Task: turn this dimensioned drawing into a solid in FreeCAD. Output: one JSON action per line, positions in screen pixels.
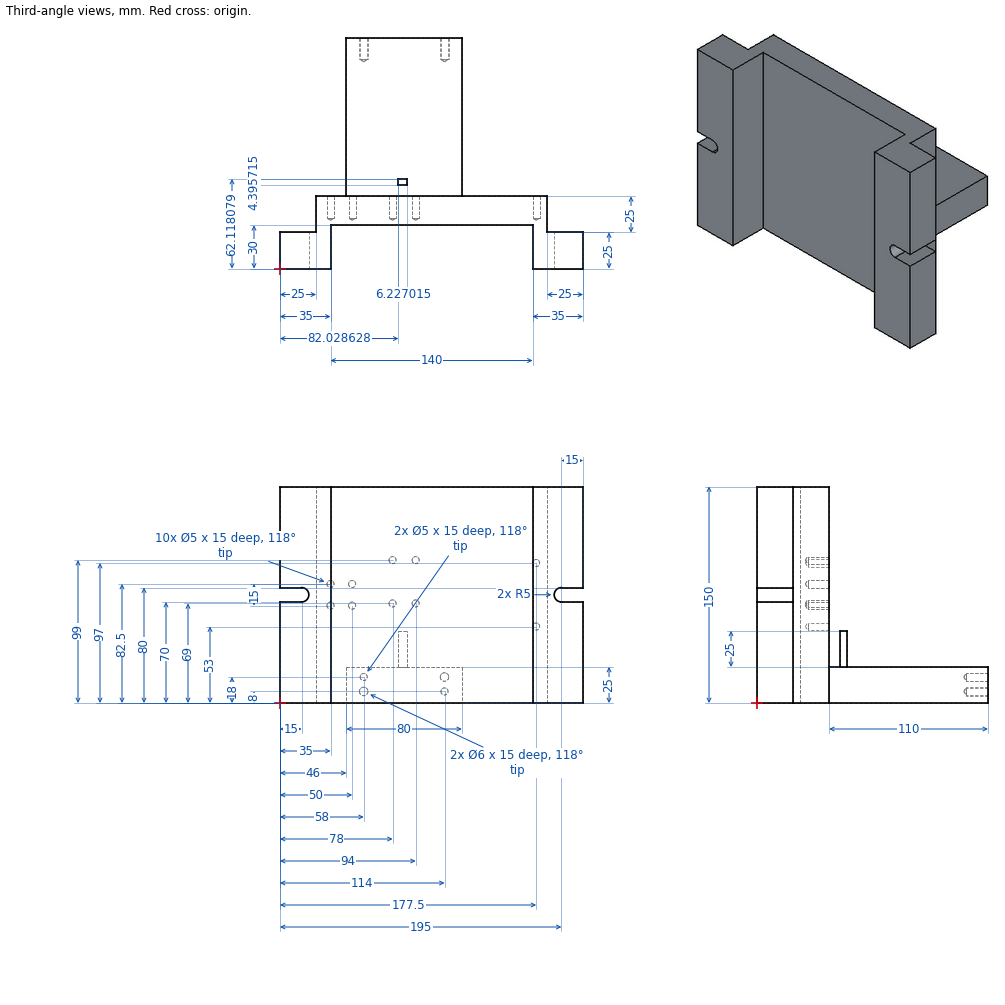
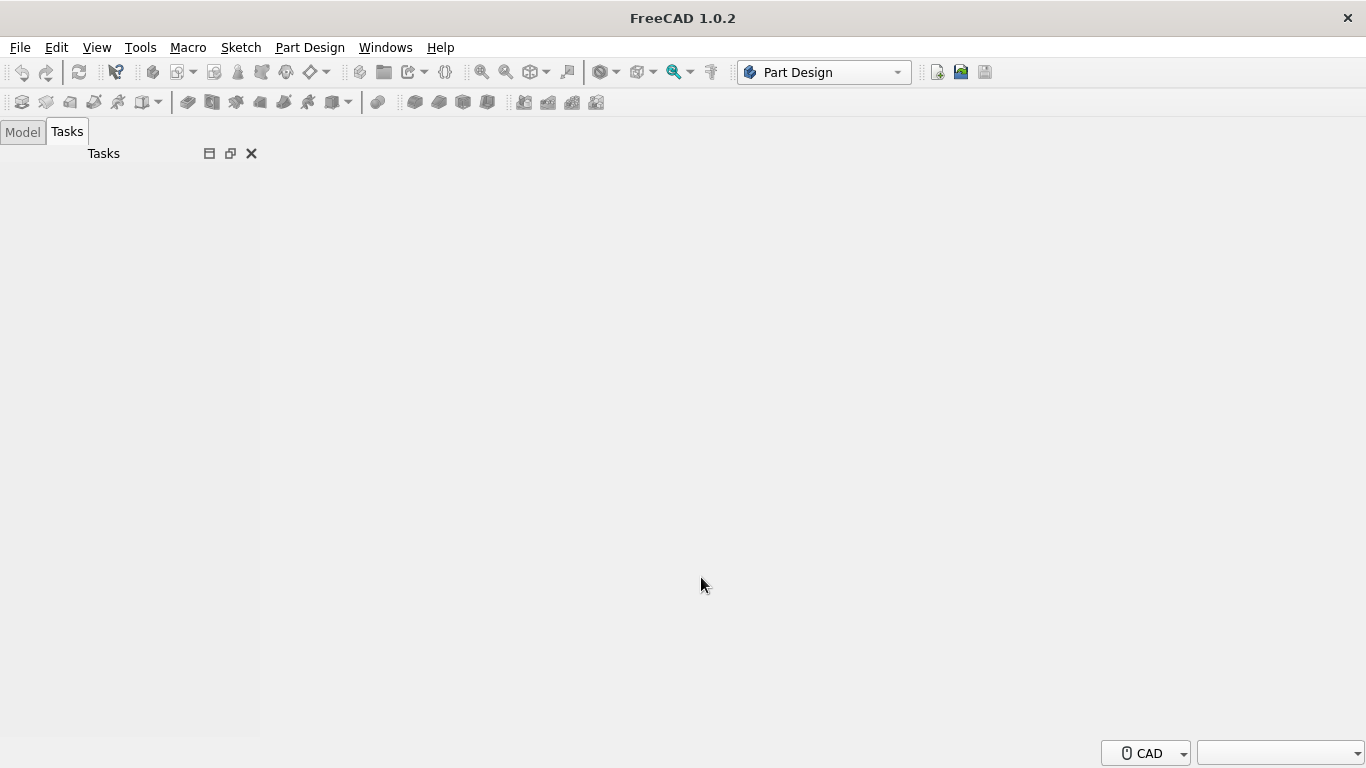
{"action": "key", "text": "ctrl+n"}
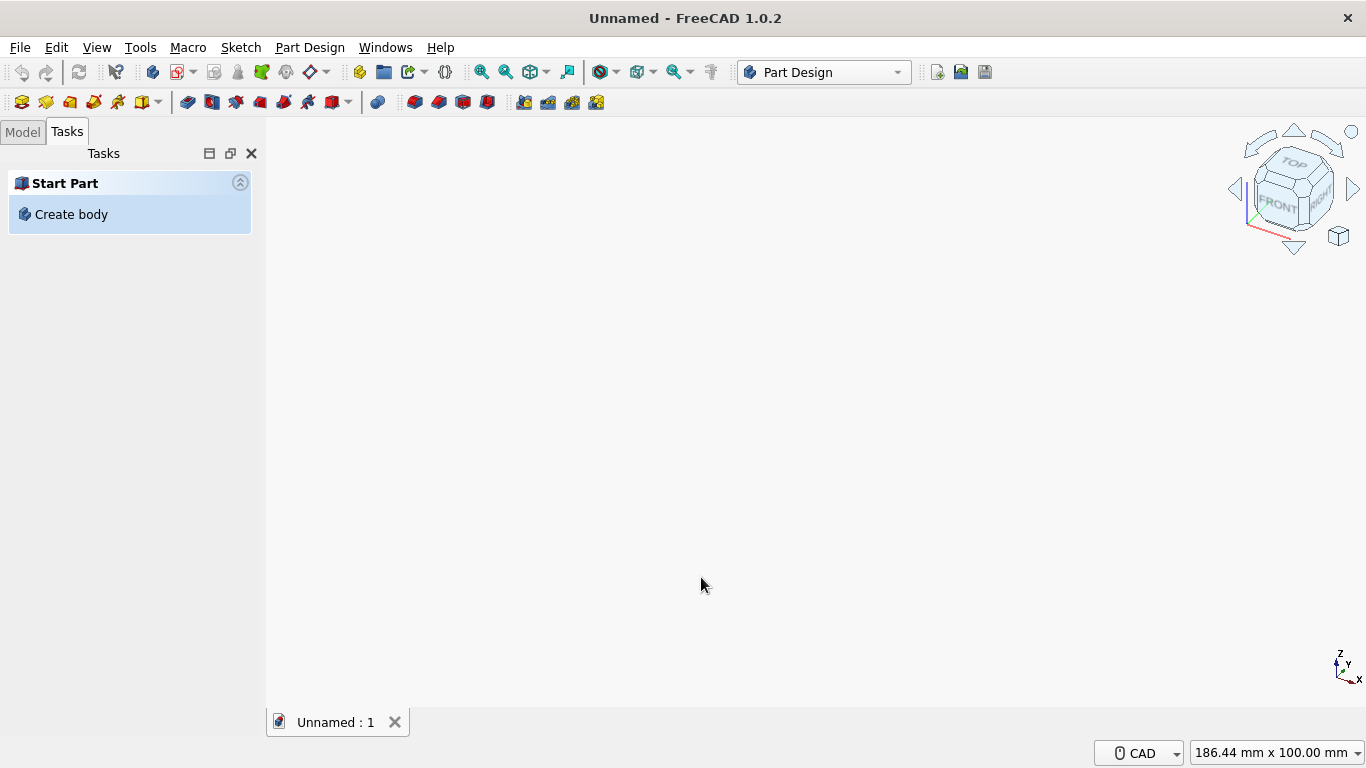
{"action": "left_click", "coordinate": [178, 72]}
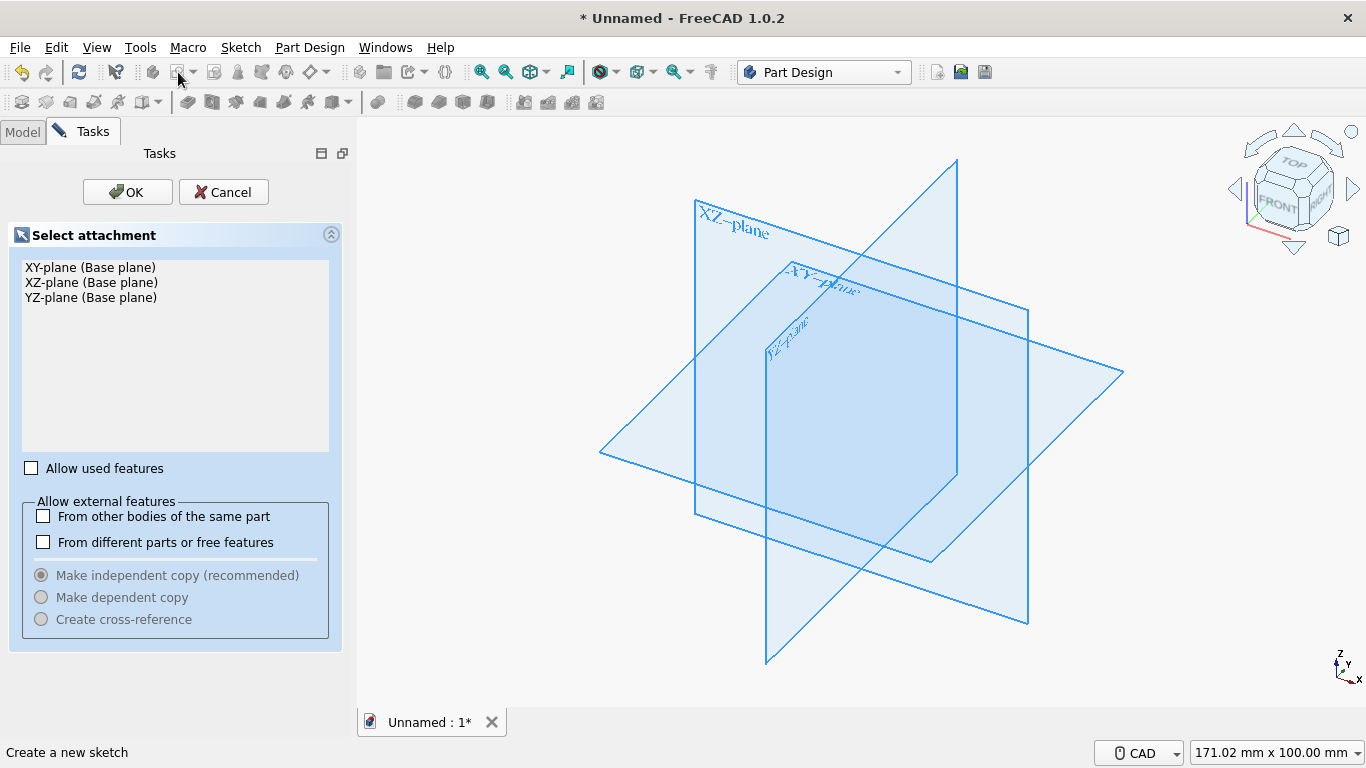
{"action": "left_click", "coordinate": [82, 268]}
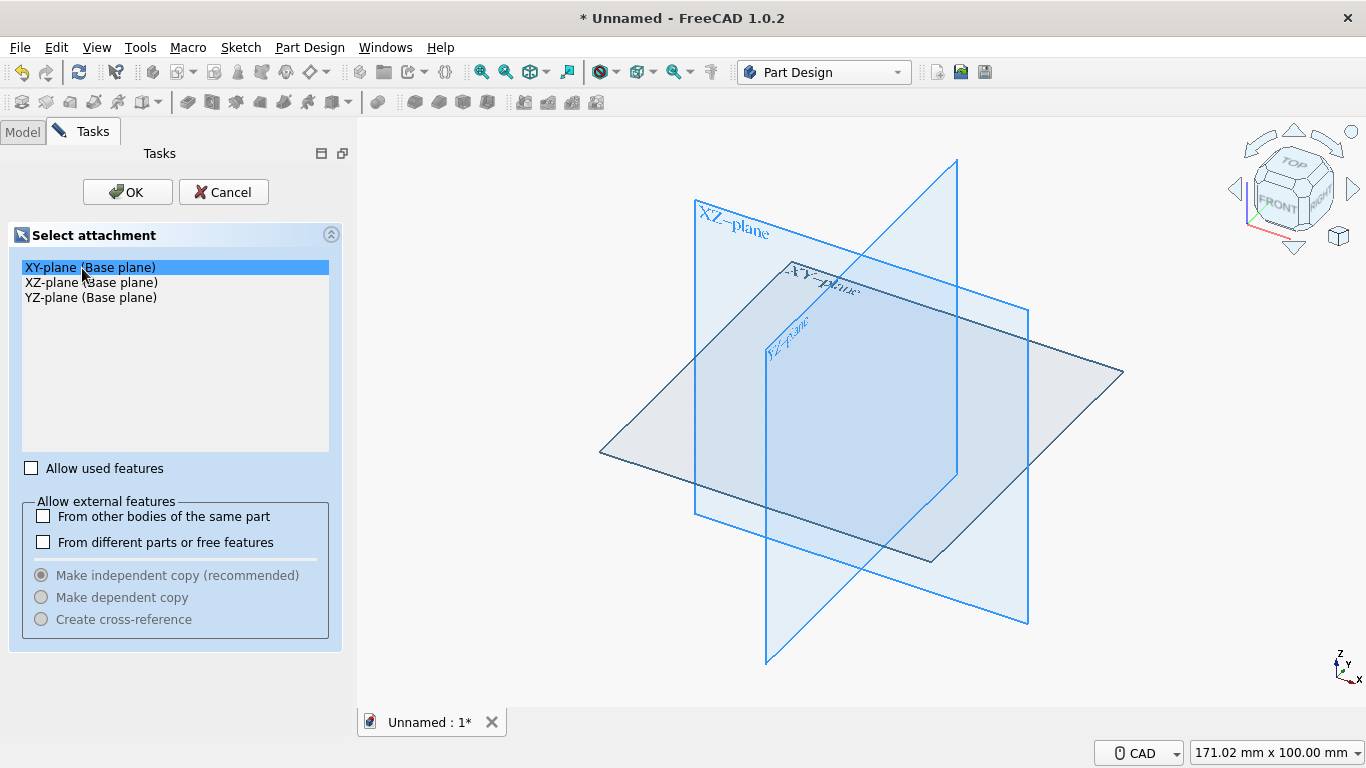
{"action": "left_click", "coordinate": [128, 192]}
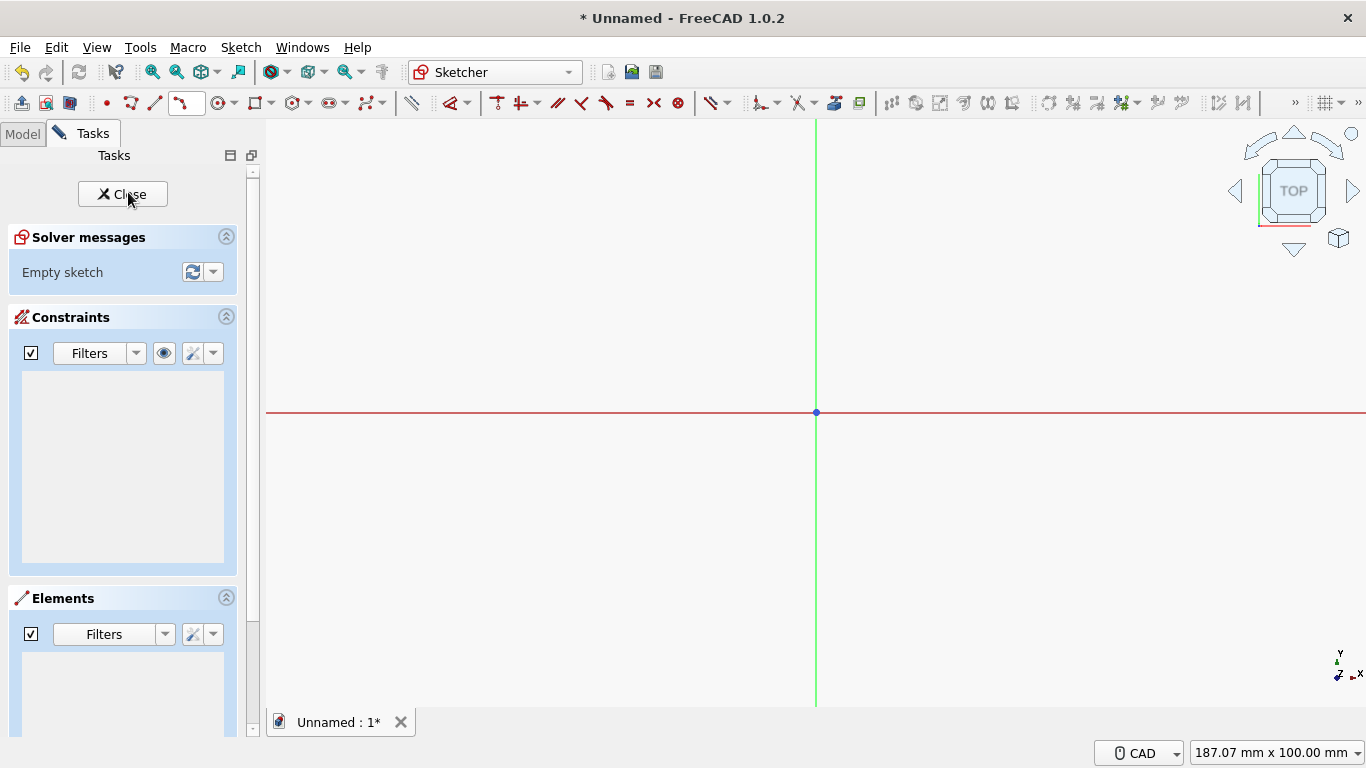
{"action": "scroll", "coordinate": [294, 533], "scroll_direction": "down", "scroll_amount": 4}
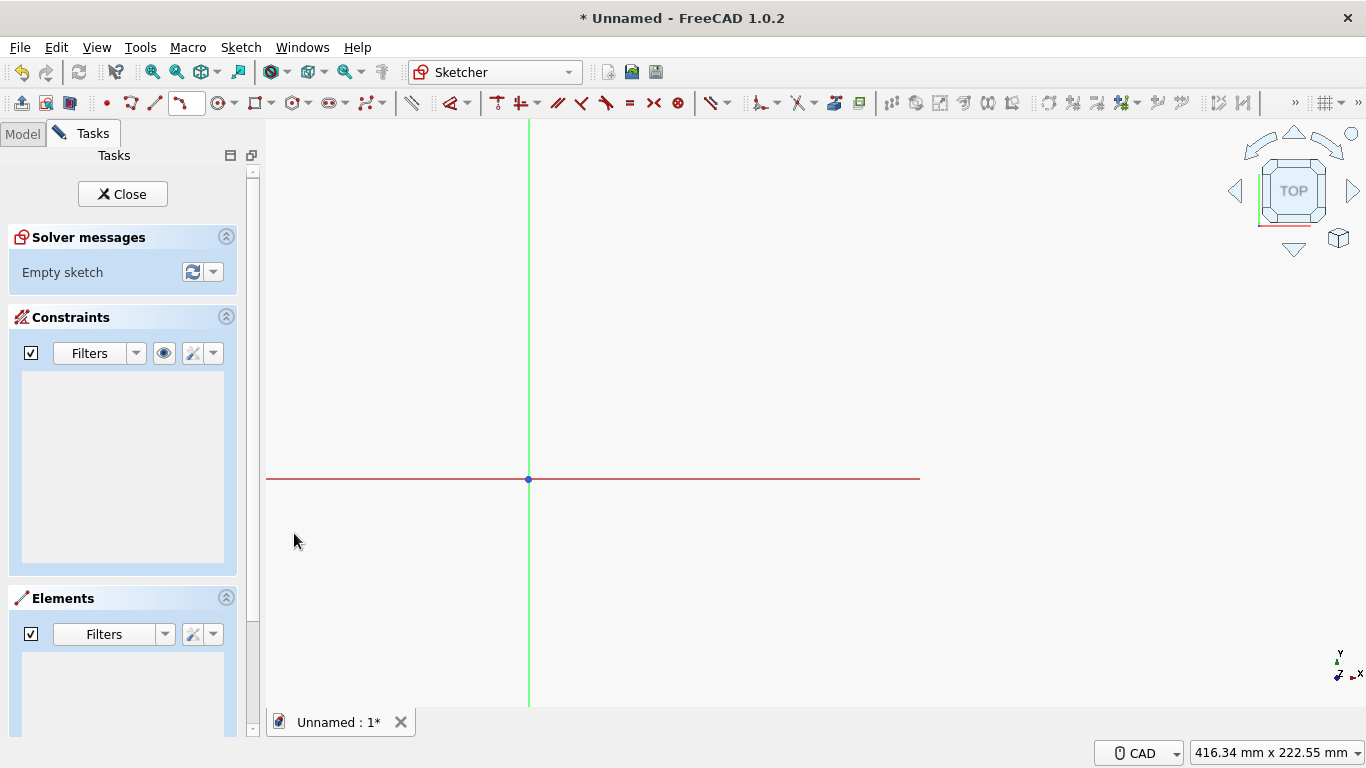
{"action": "key", "text": "g m"}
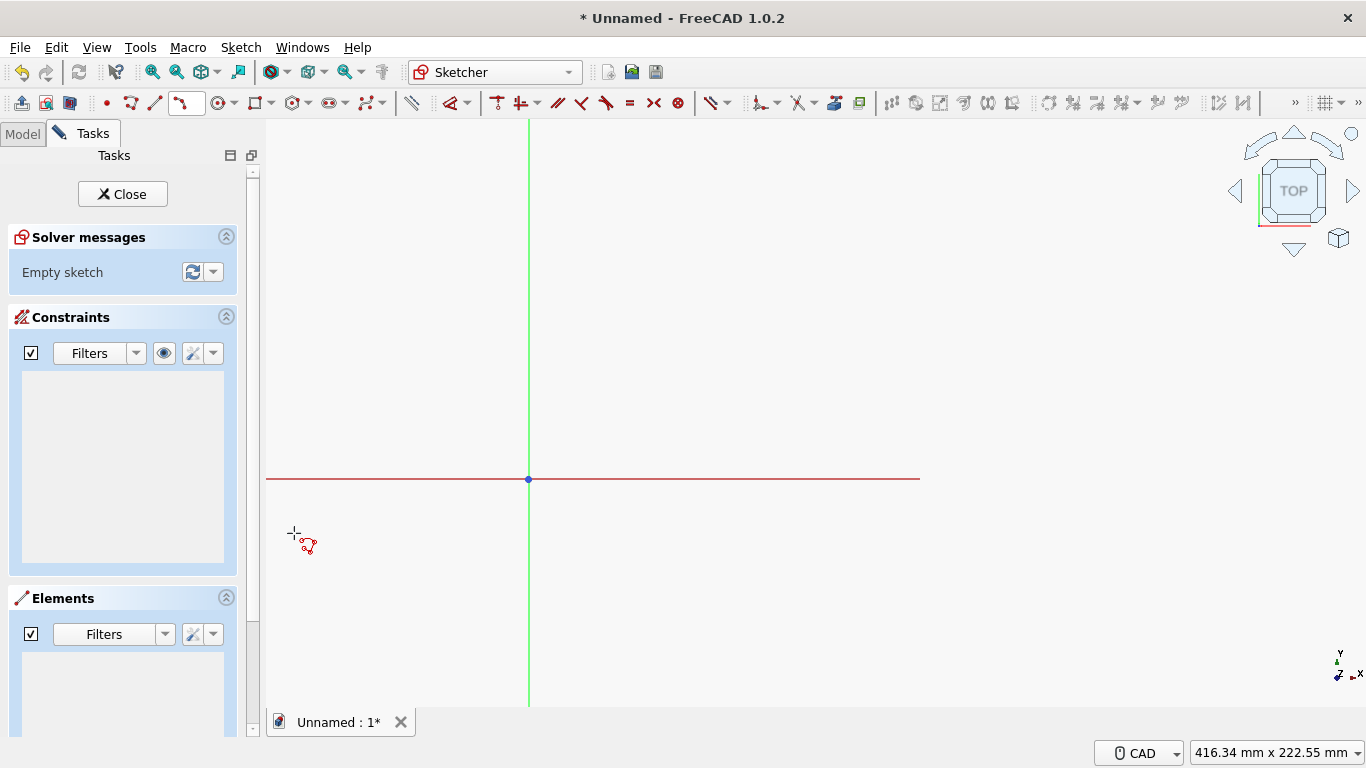
{"action": "left_click", "coordinate": [529, 479]}
{"action": "left_click", "coordinate": [621, 470]}
{"action": "left_click", "coordinate": [621, 400]}
{"action": "left_click", "coordinate": [991, 400]}
{"action": "left_click", "coordinate": [991, 479]}
{"action": "left_click", "coordinate": [1083, 470]}
{"action": "left_click", "coordinate": [1083, 413]}
{"action": "left_click", "coordinate": [1017, 413]}
{"action": "left_click", "coordinate": [1017, 347]}
{"action": "left_click", "coordinate": [595, 347]}
{"action": "left_click", "coordinate": [595, 413]}
{"action": "left_click", "coordinate": [538, 413]}
{"action": "left_click", "coordinate": [529, 479]}
{"action": "key", "text": "Escape"}
{"action": "key", "text": "Escape"}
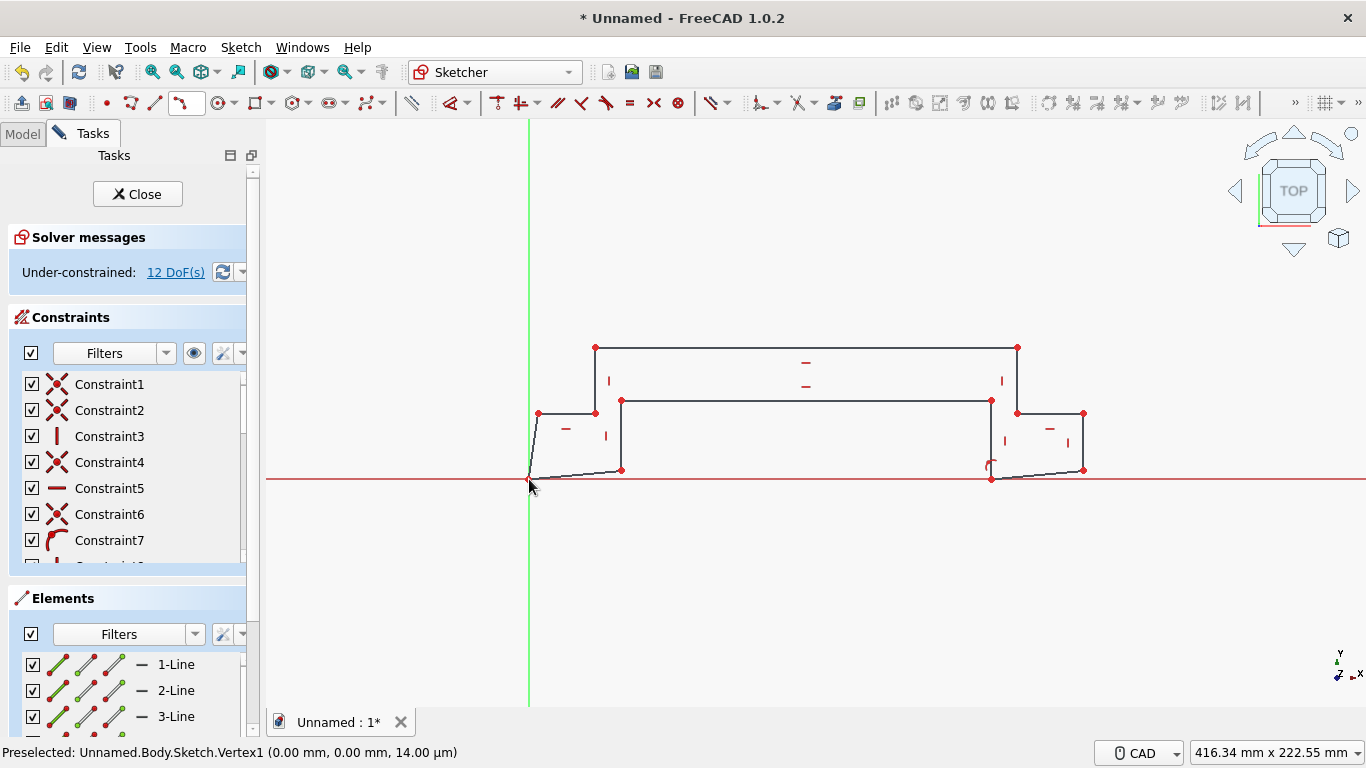
{"action": "left_click", "coordinate": [556, 477]}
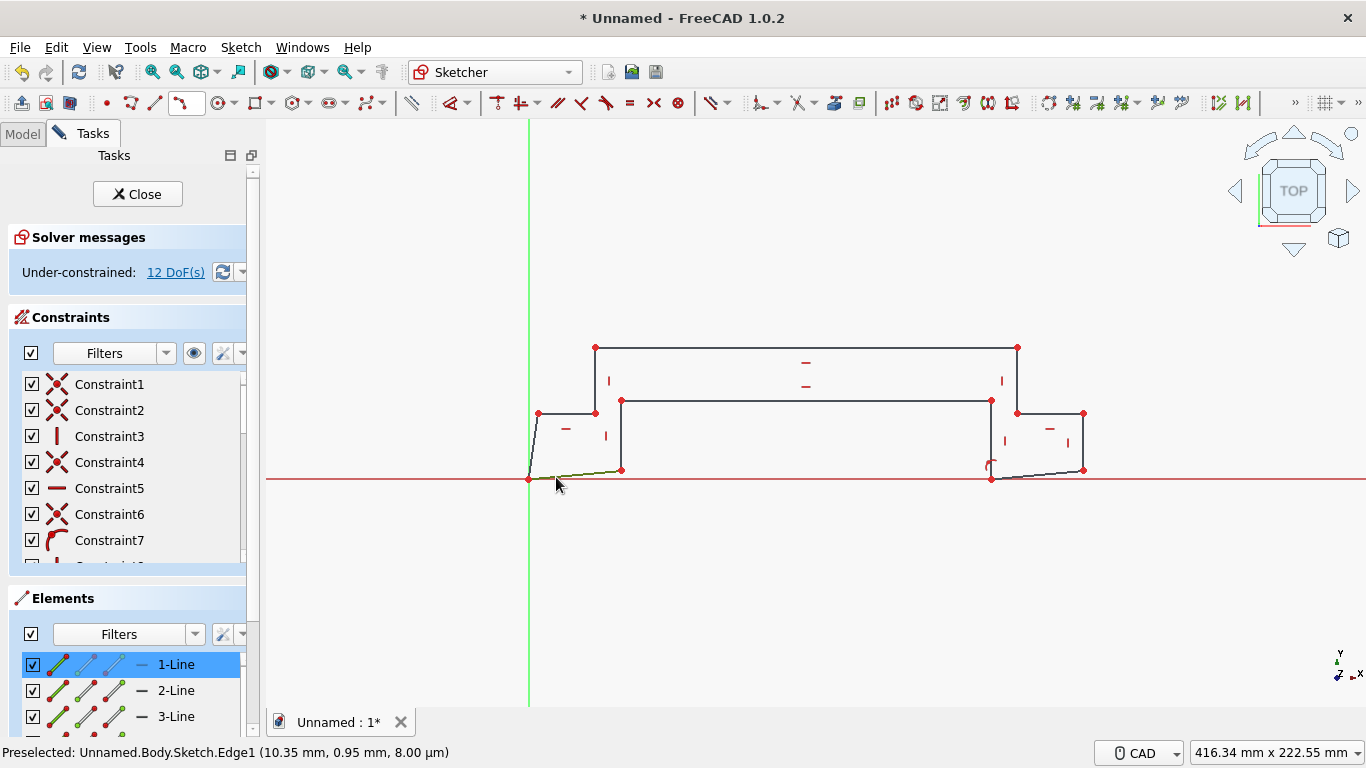
{"action": "key", "text": "h"}